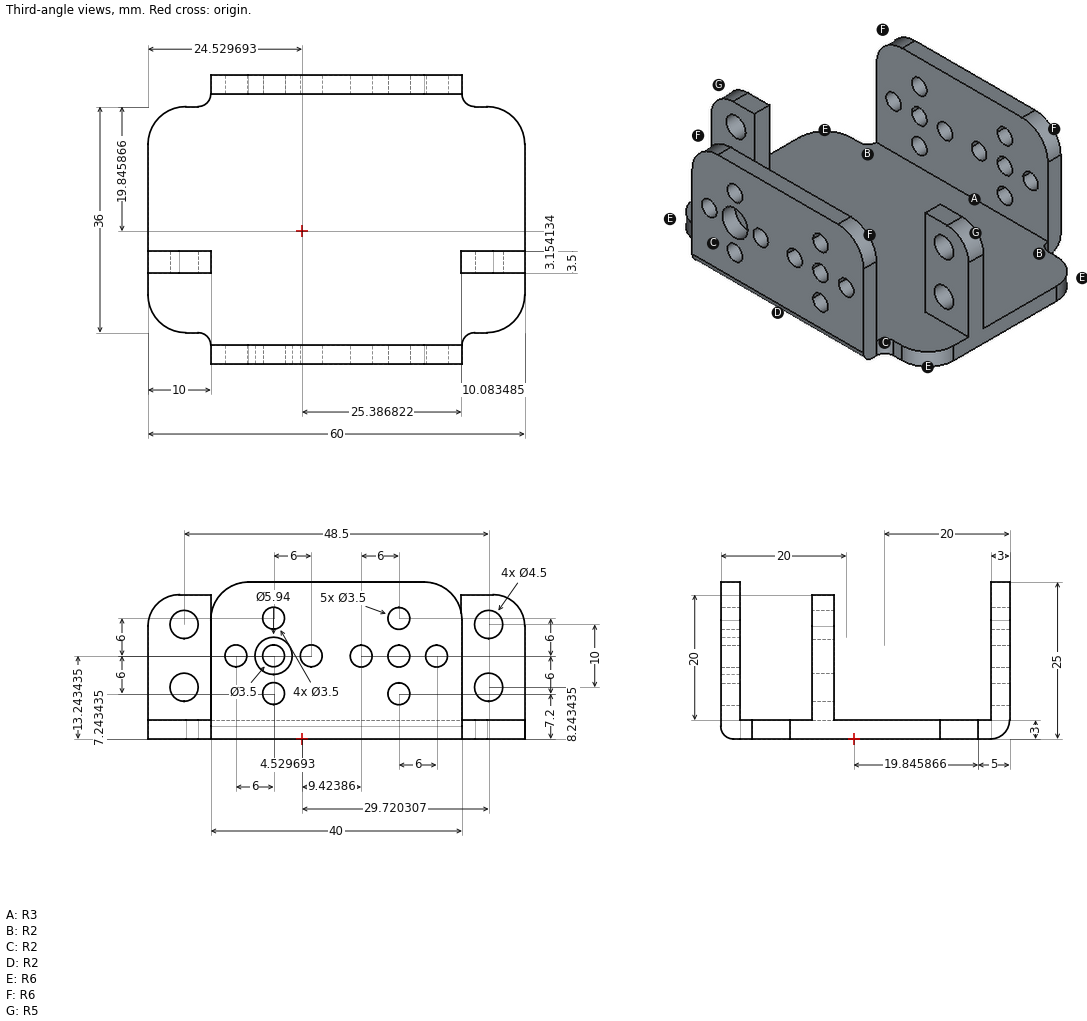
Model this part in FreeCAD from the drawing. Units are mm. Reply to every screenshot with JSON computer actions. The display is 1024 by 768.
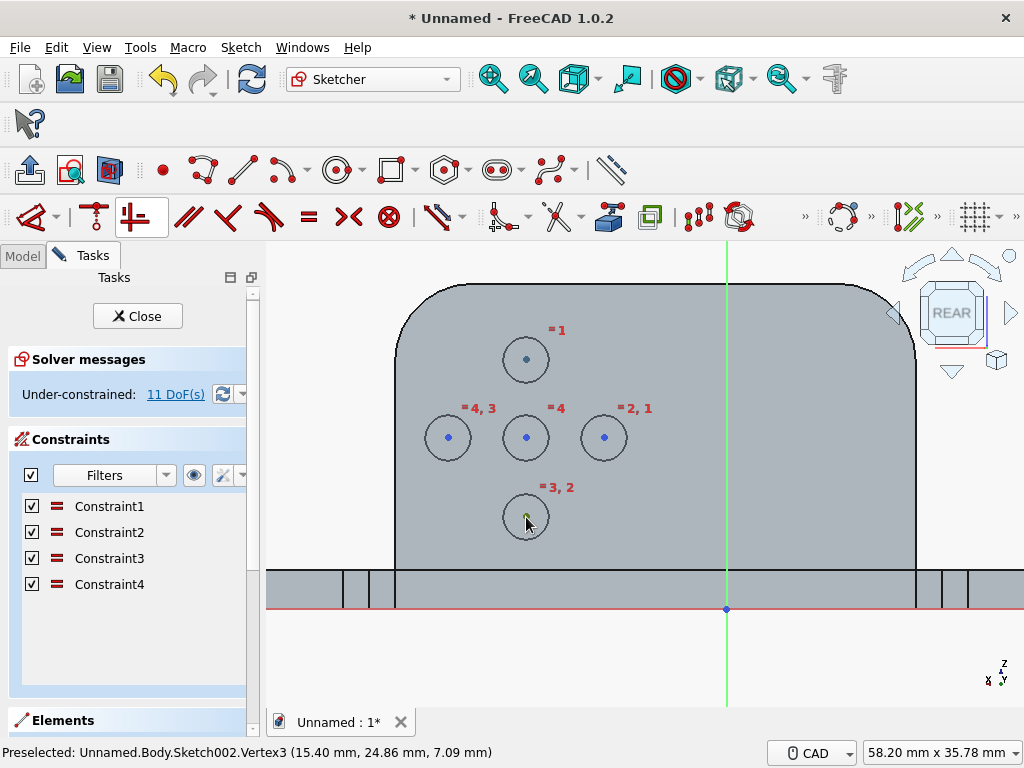
{"action": "key", "text": "v"}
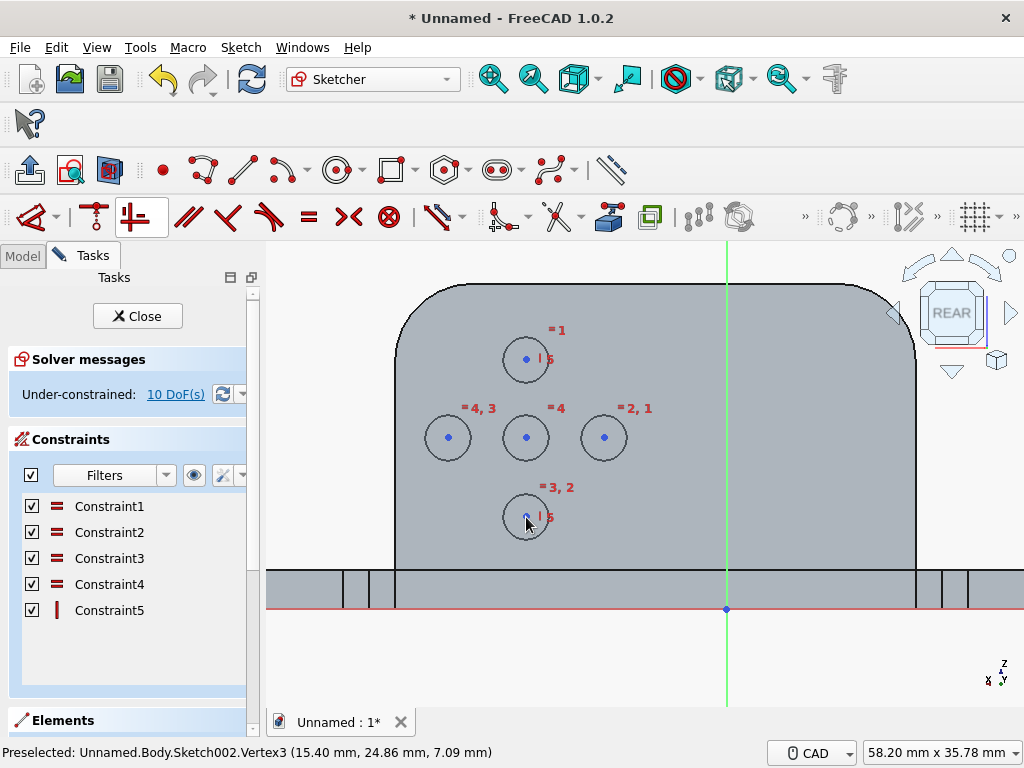
{"action": "left_click", "coordinate": [604, 438]}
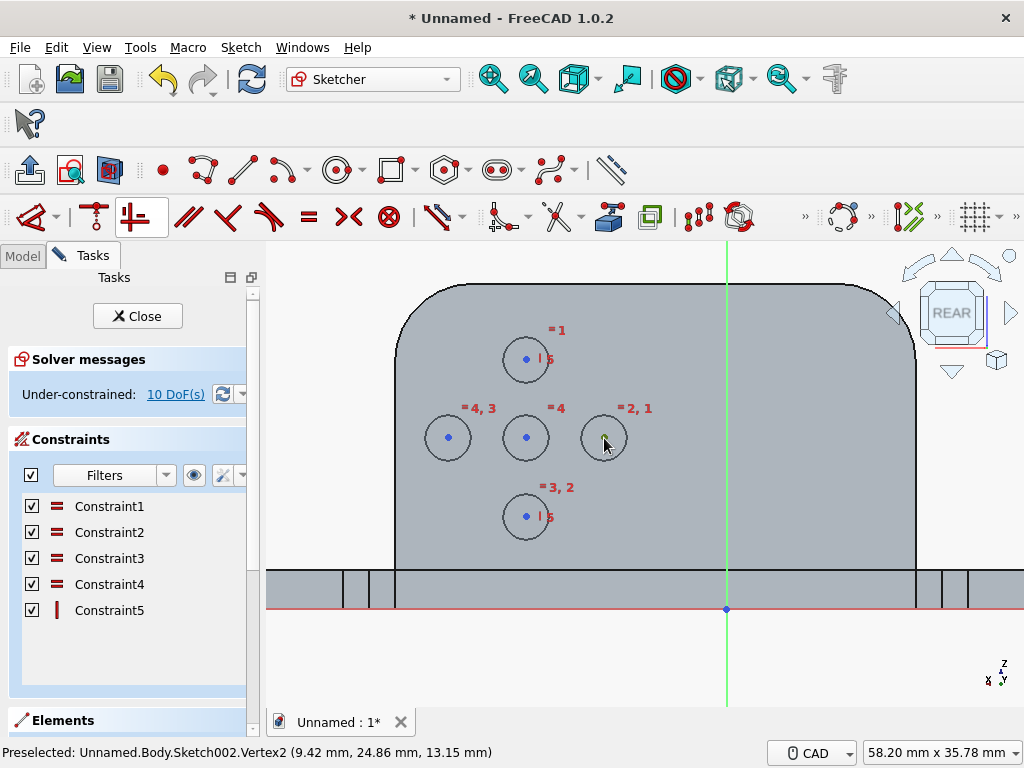
{"action": "left_click", "coordinate": [448, 438]}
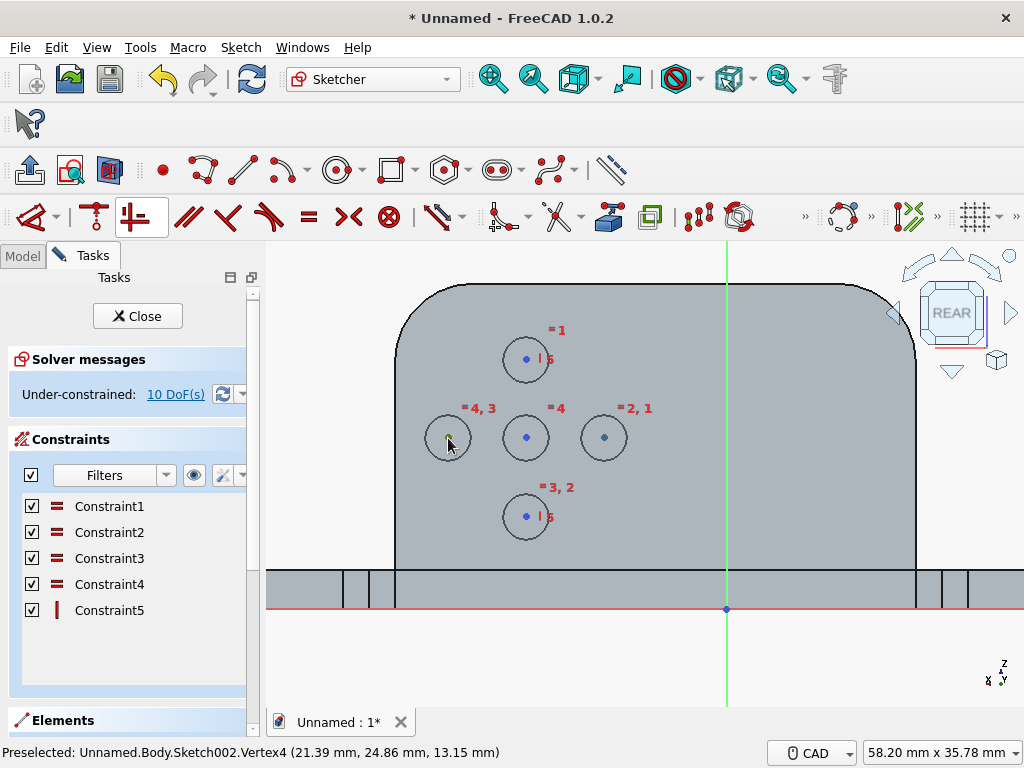
{"action": "left_click", "coordinate": [162, 218]}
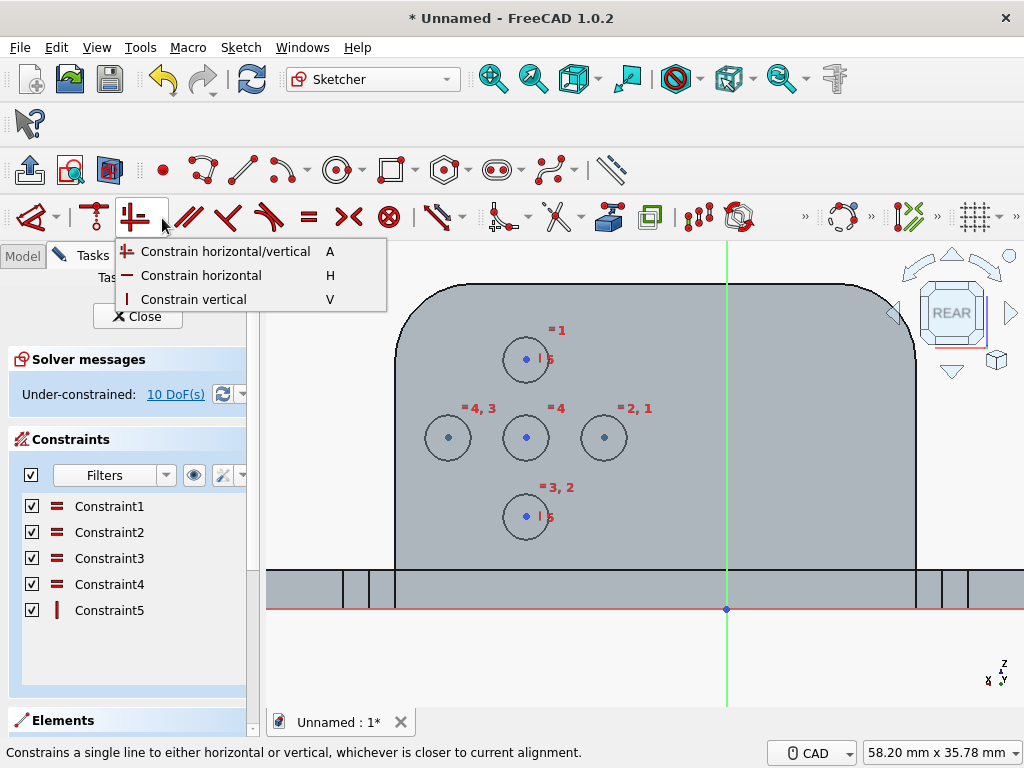
{"action": "left_click", "coordinate": [251, 275]}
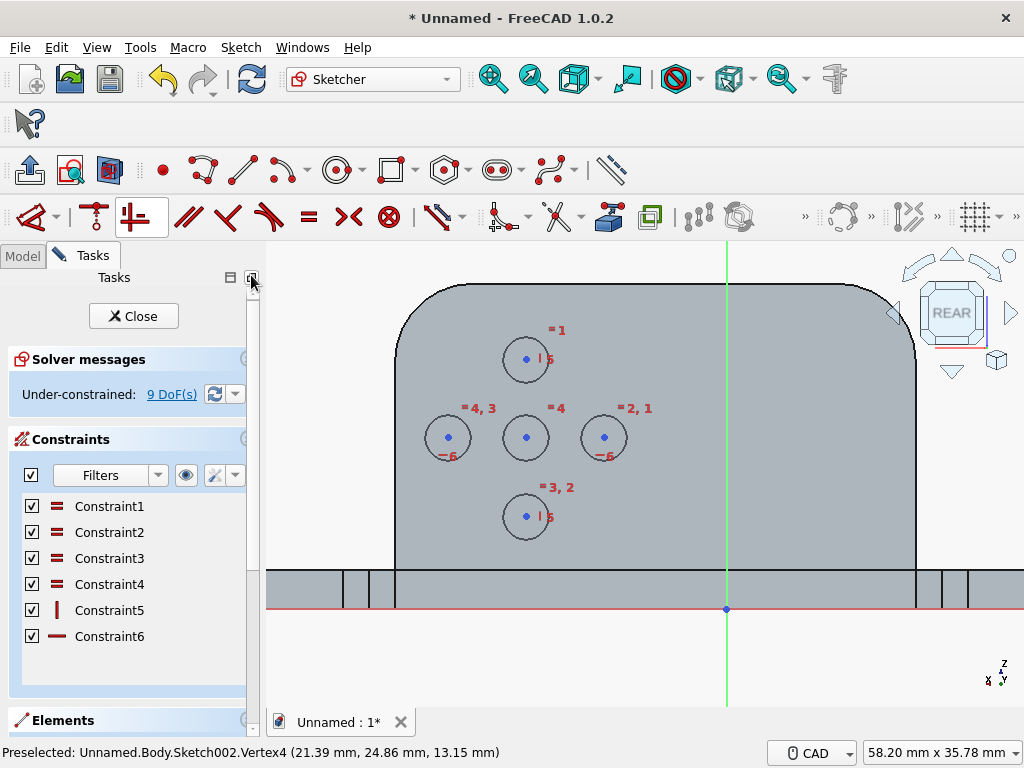
{"action": "left_click", "coordinate": [526, 517]}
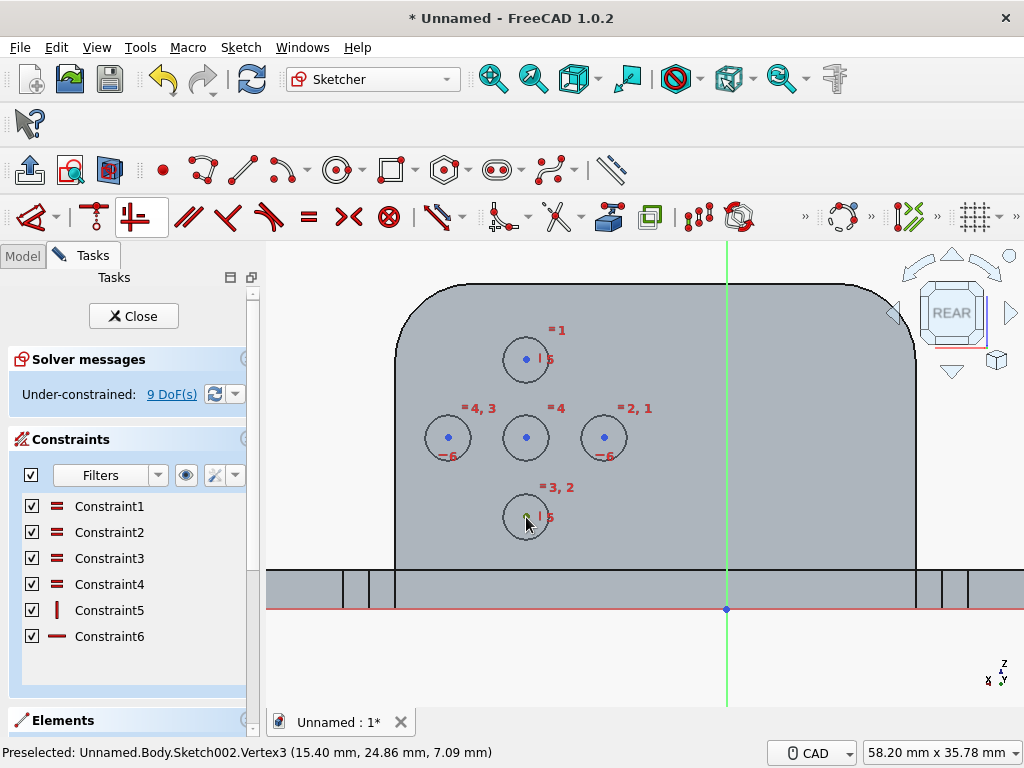
{"action": "left_click", "coordinate": [526, 438]}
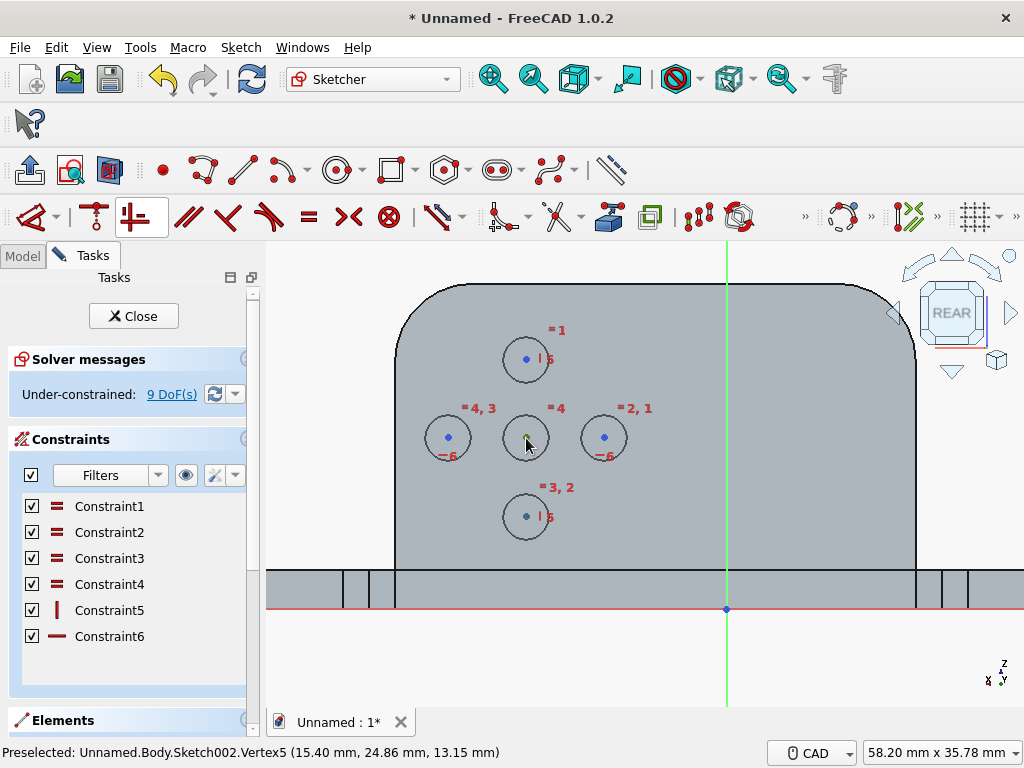
{"action": "left_click", "coordinate": [162, 218]}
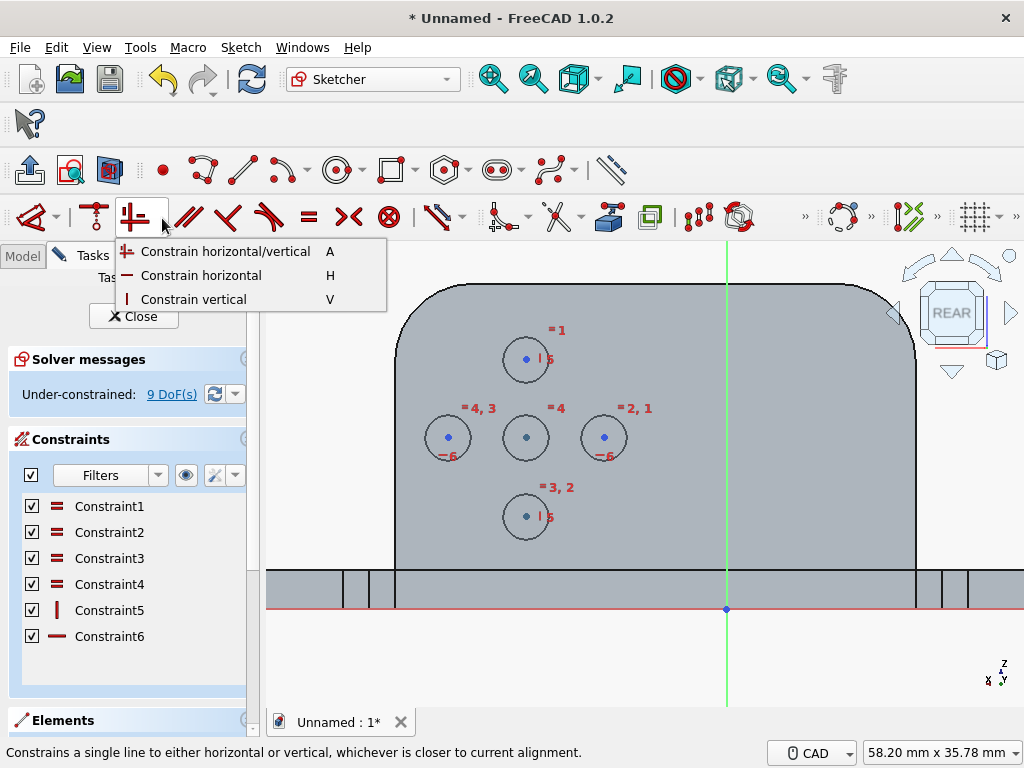
{"action": "left_click", "coordinate": [251, 299]}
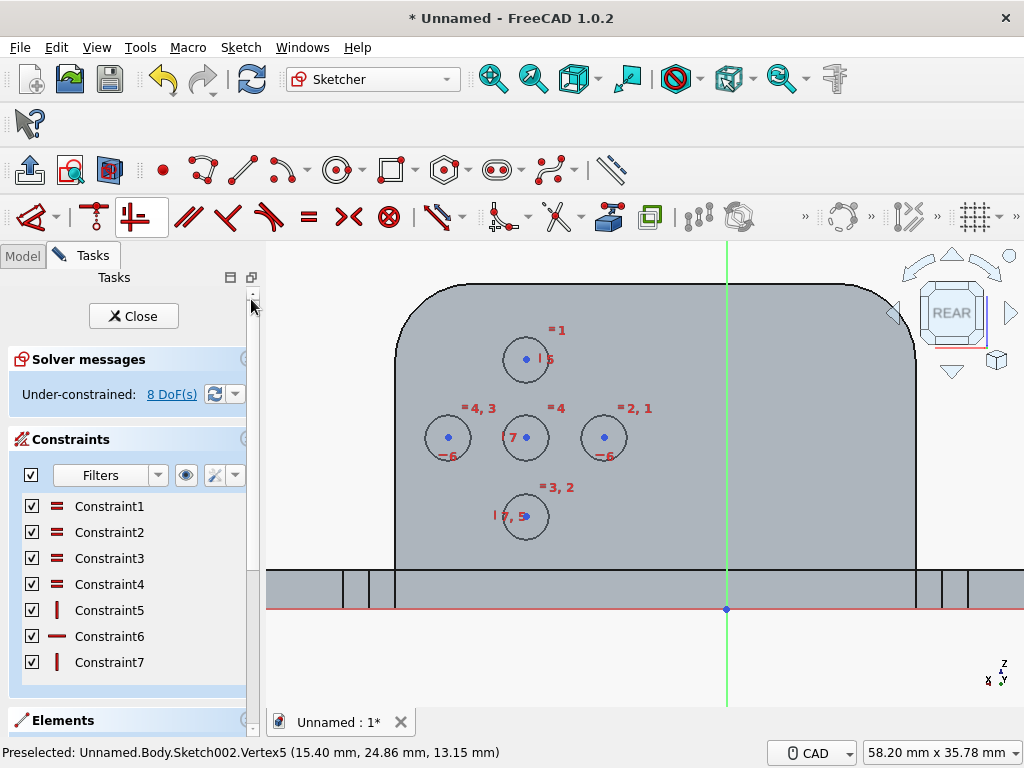
{"action": "left_click", "coordinate": [448, 438]}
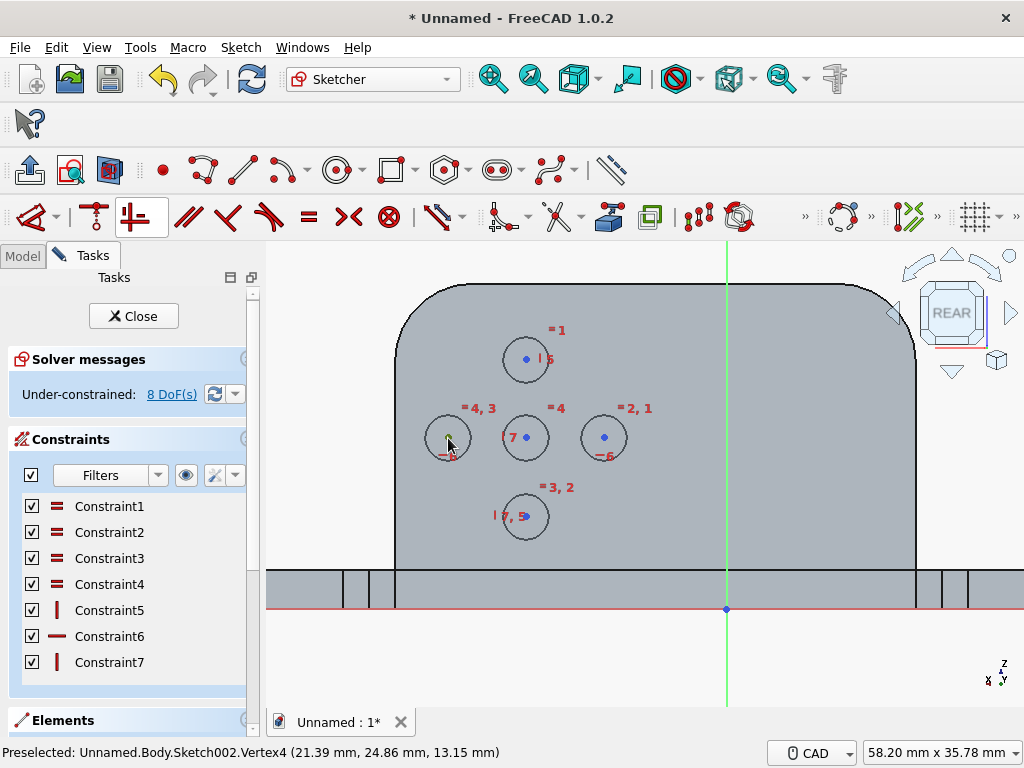
{"action": "left_click", "coordinate": [526, 438]}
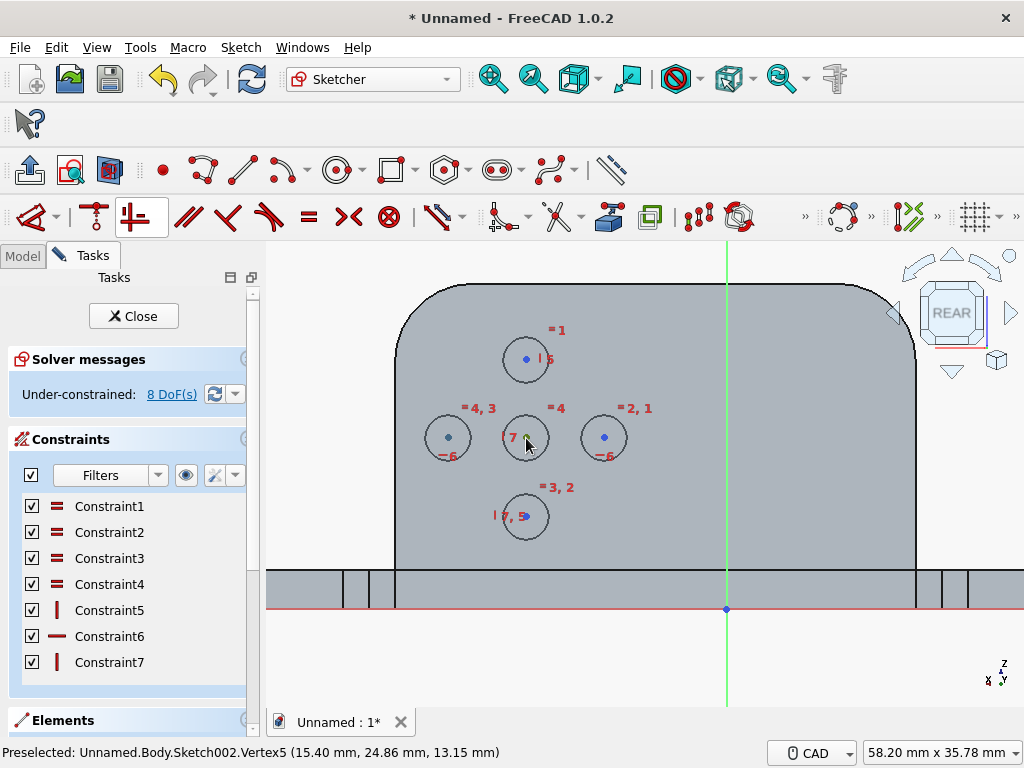
{"action": "left_click", "coordinate": [162, 218]}